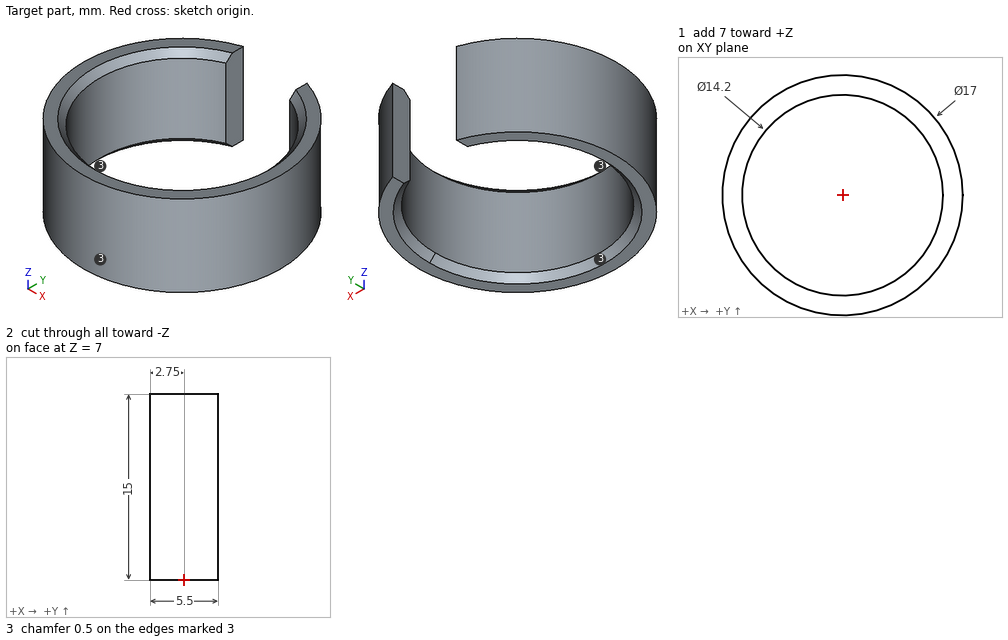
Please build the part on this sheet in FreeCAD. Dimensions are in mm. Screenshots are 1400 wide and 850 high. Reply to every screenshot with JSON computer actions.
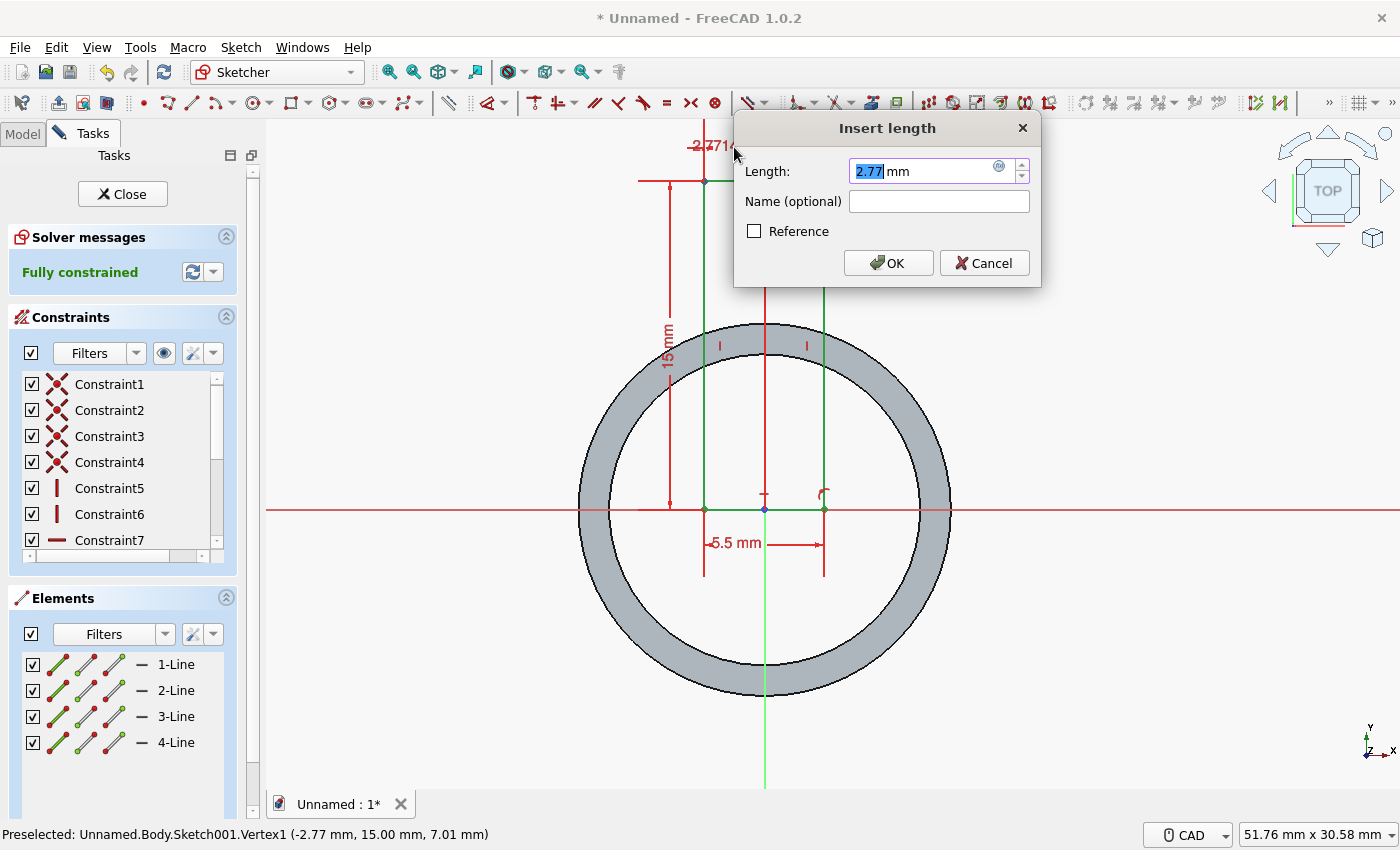
{"action": "type", "text": "2.75"}
{"action": "key", "text": "Return"}
{"action": "key", "text": "Escape"}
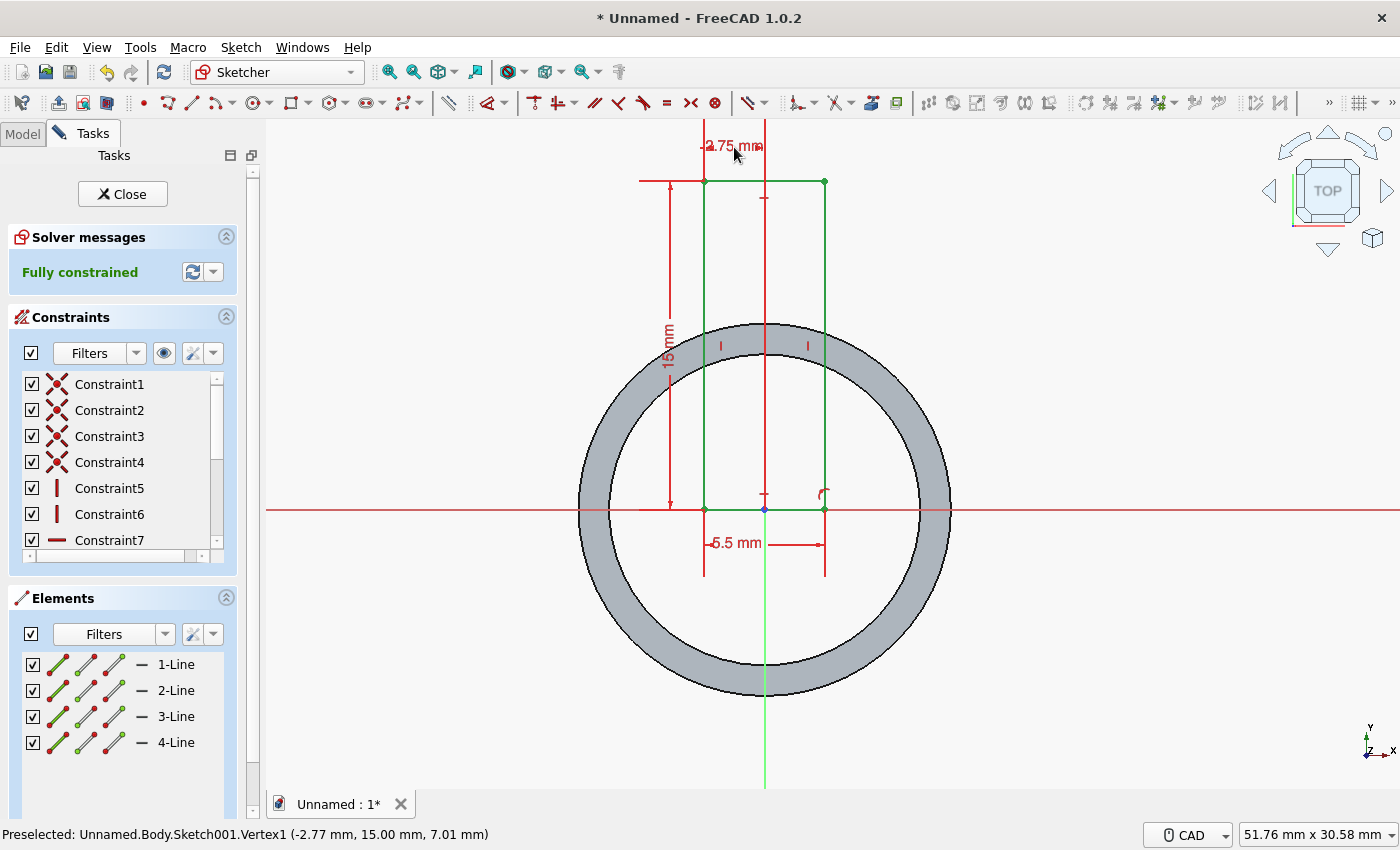
{"action": "left_click", "coordinate": [123, 194]}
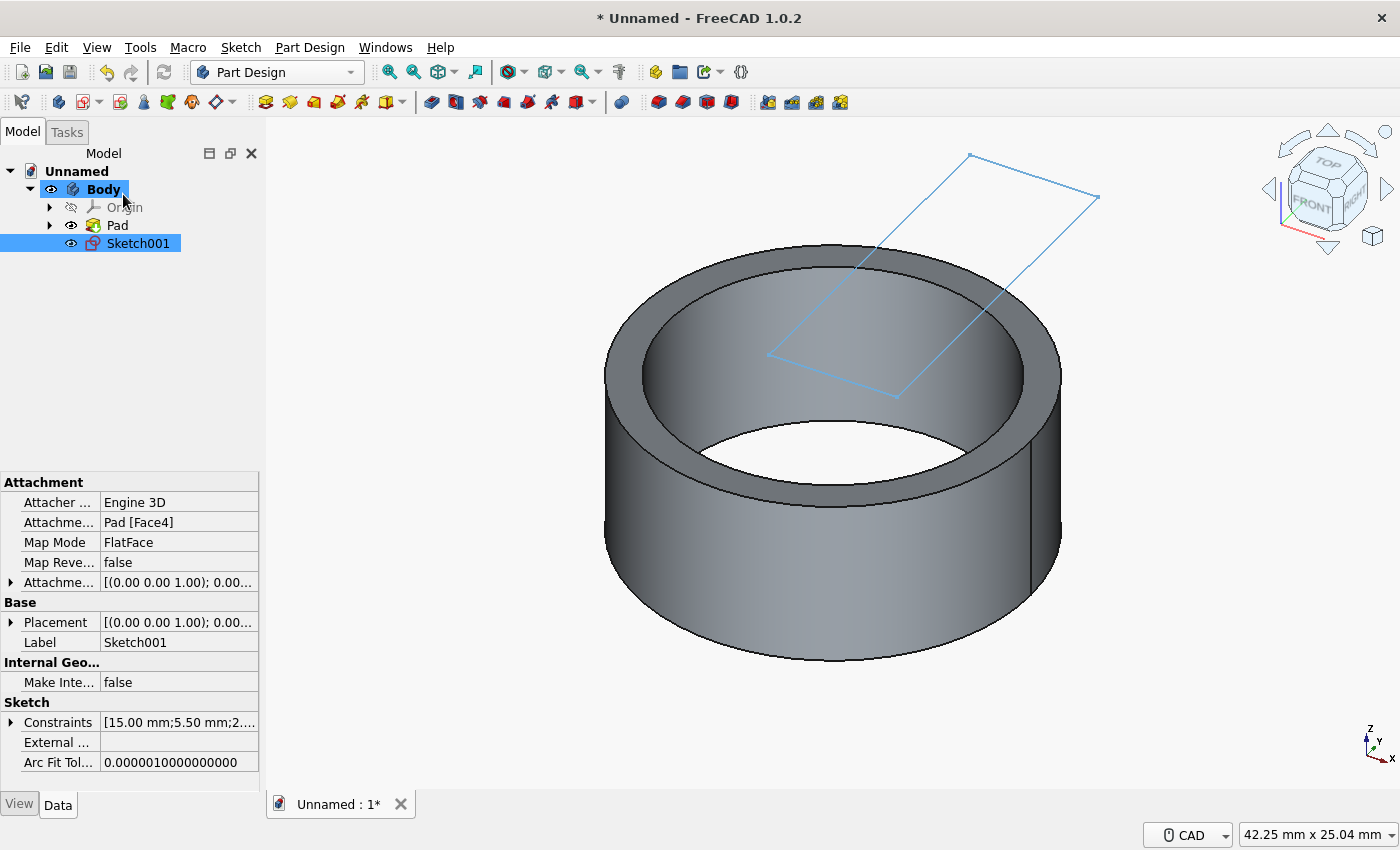
{"action": "left_click", "coordinate": [432, 102]}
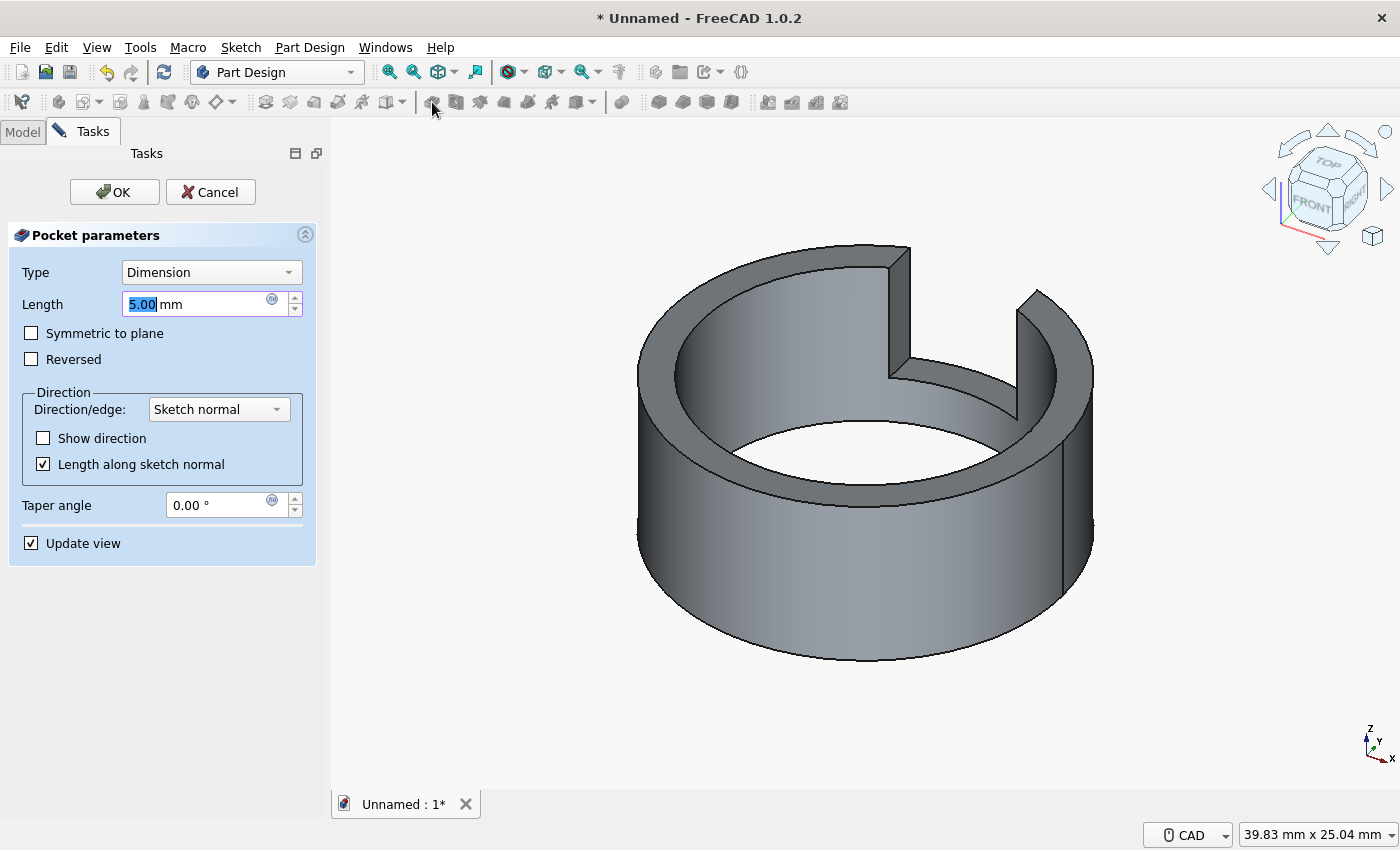
{"action": "left_click", "coordinate": [212, 272]}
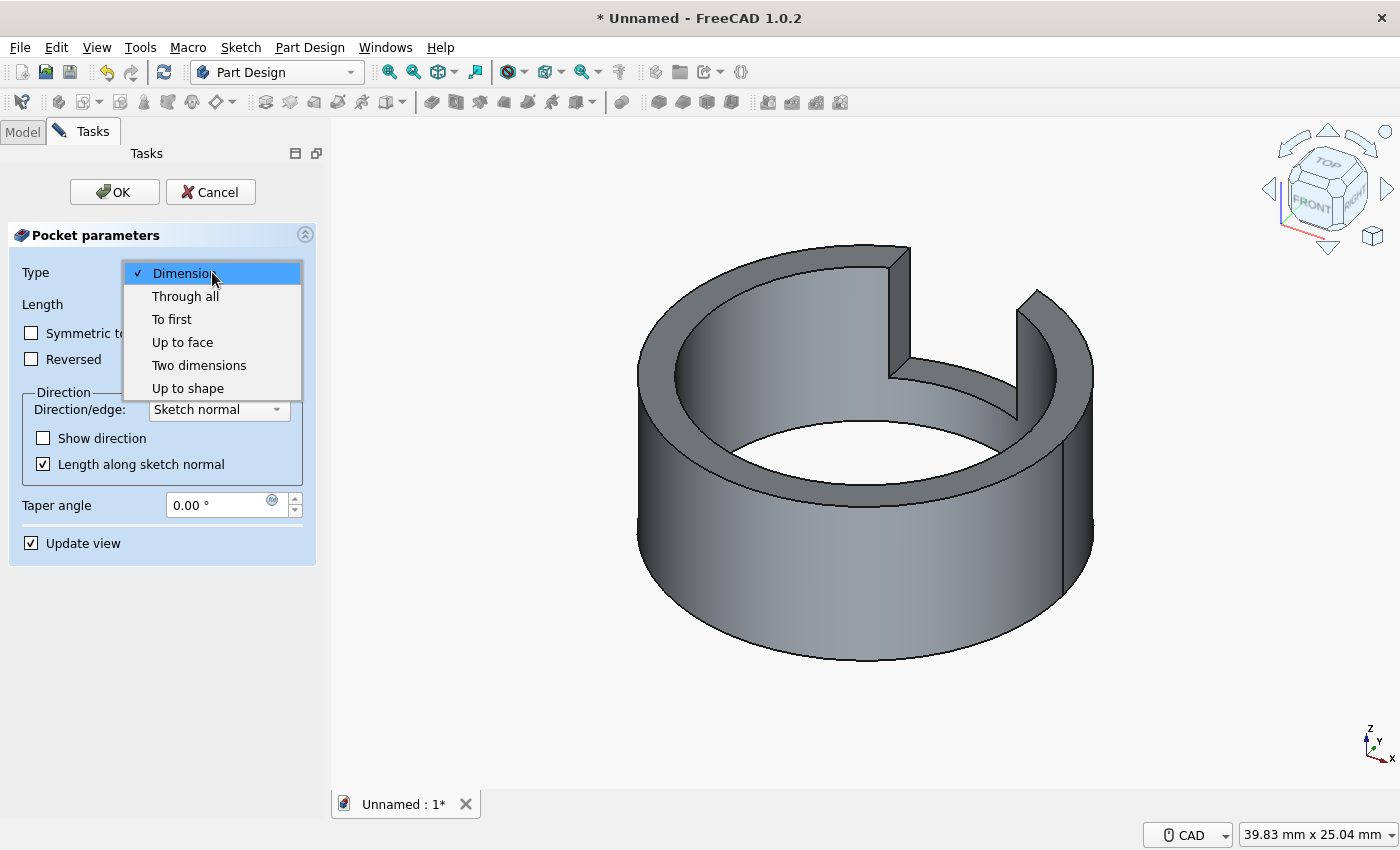
{"action": "left_click", "coordinate": [212, 296]}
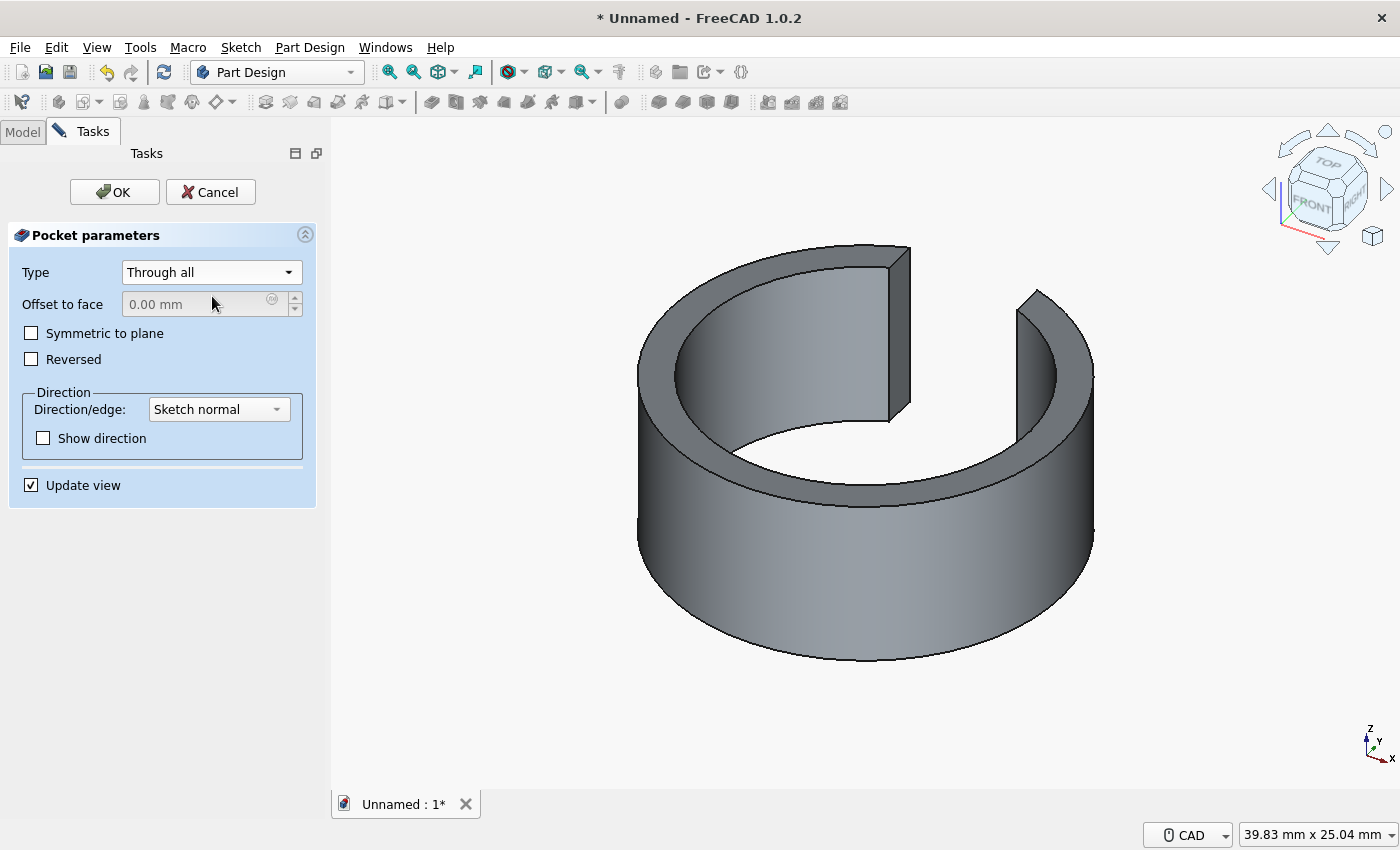
{"action": "left_click", "coordinate": [115, 192]}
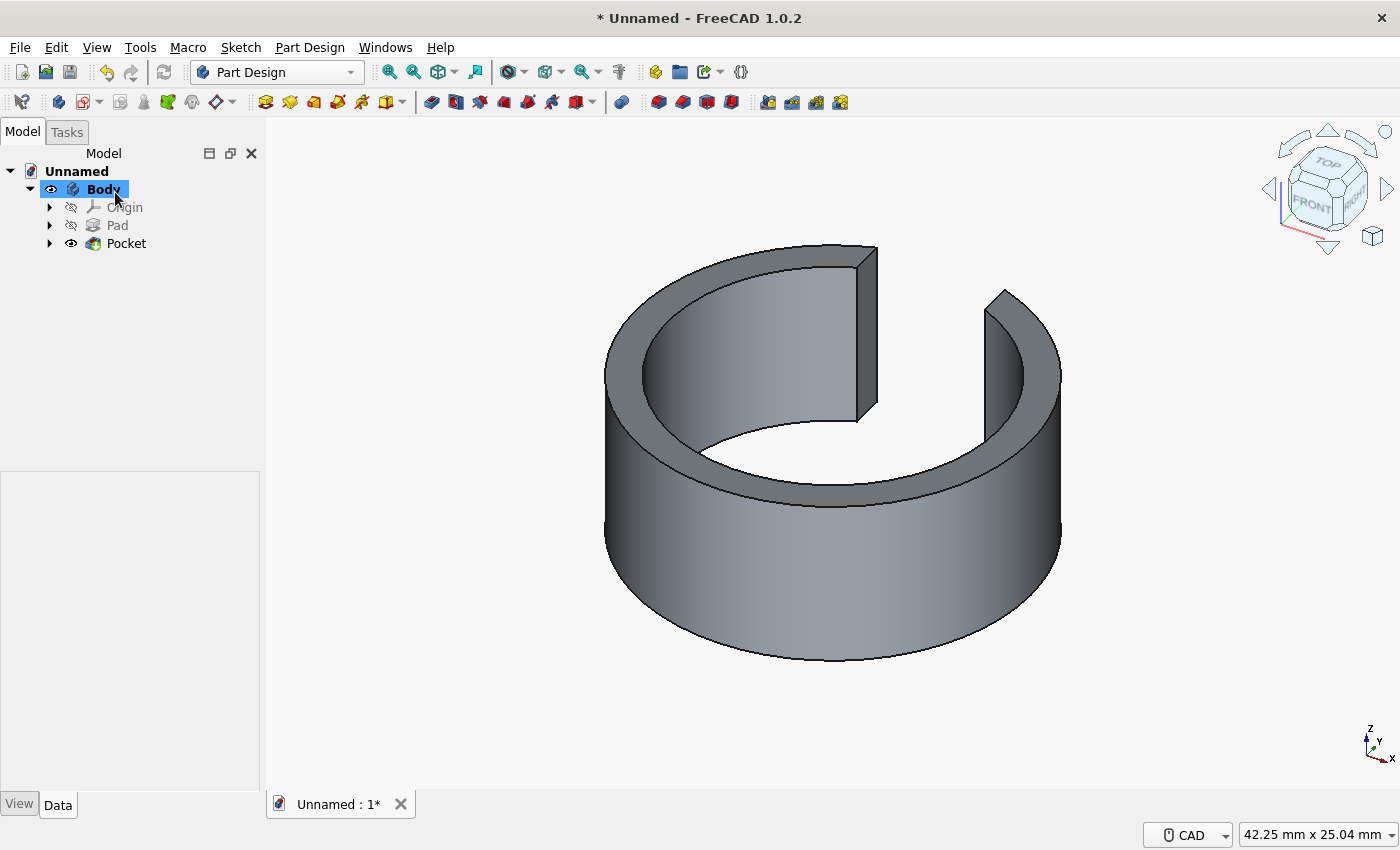
{"action": "left_click", "coordinate": [658, 332]}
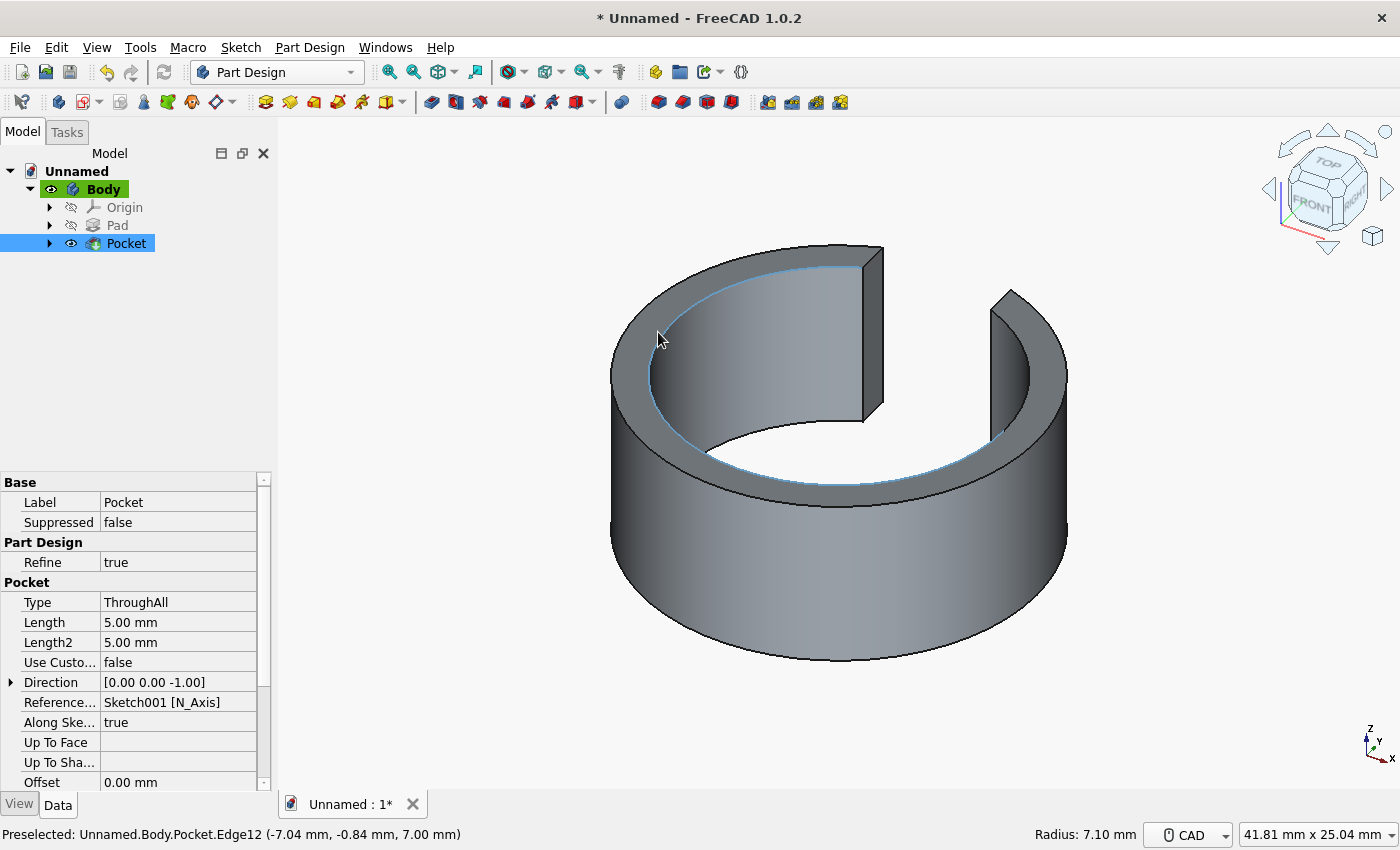
{"action": "key", "text": "0"}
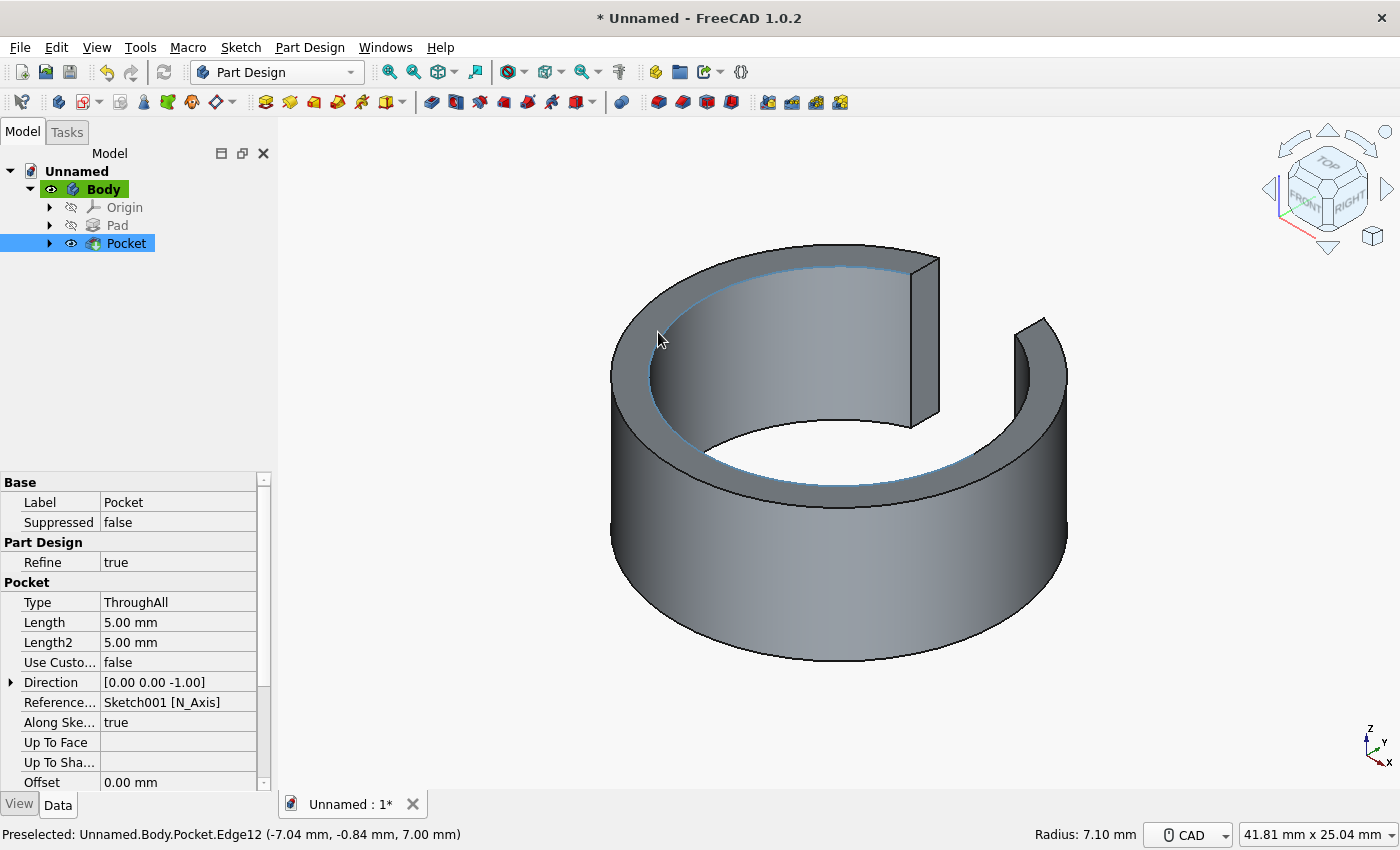
{"action": "key", "text": "2"}